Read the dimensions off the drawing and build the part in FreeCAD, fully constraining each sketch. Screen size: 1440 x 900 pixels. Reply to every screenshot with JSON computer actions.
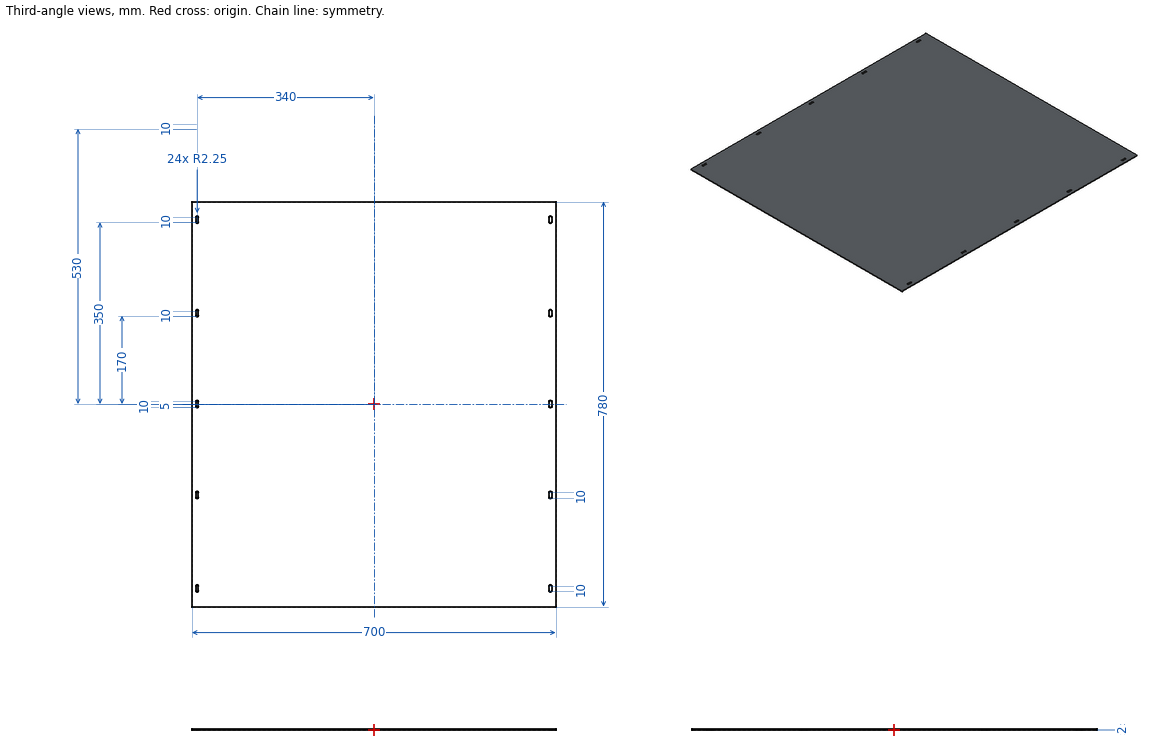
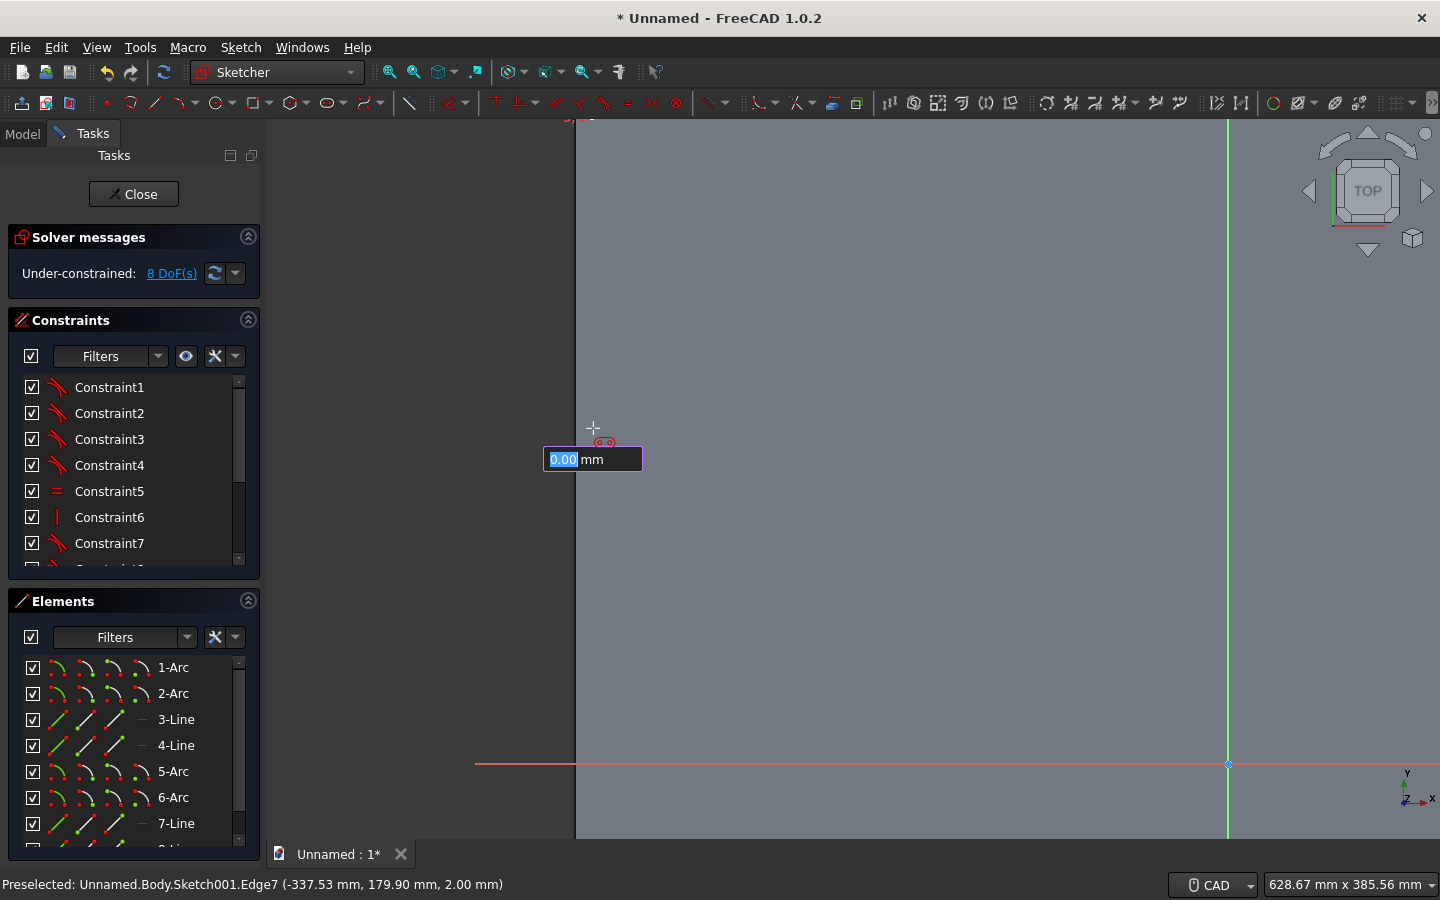
{"action": "scroll", "coordinate": [589, 437], "scroll_direction": "up", "scroll_amount": 7}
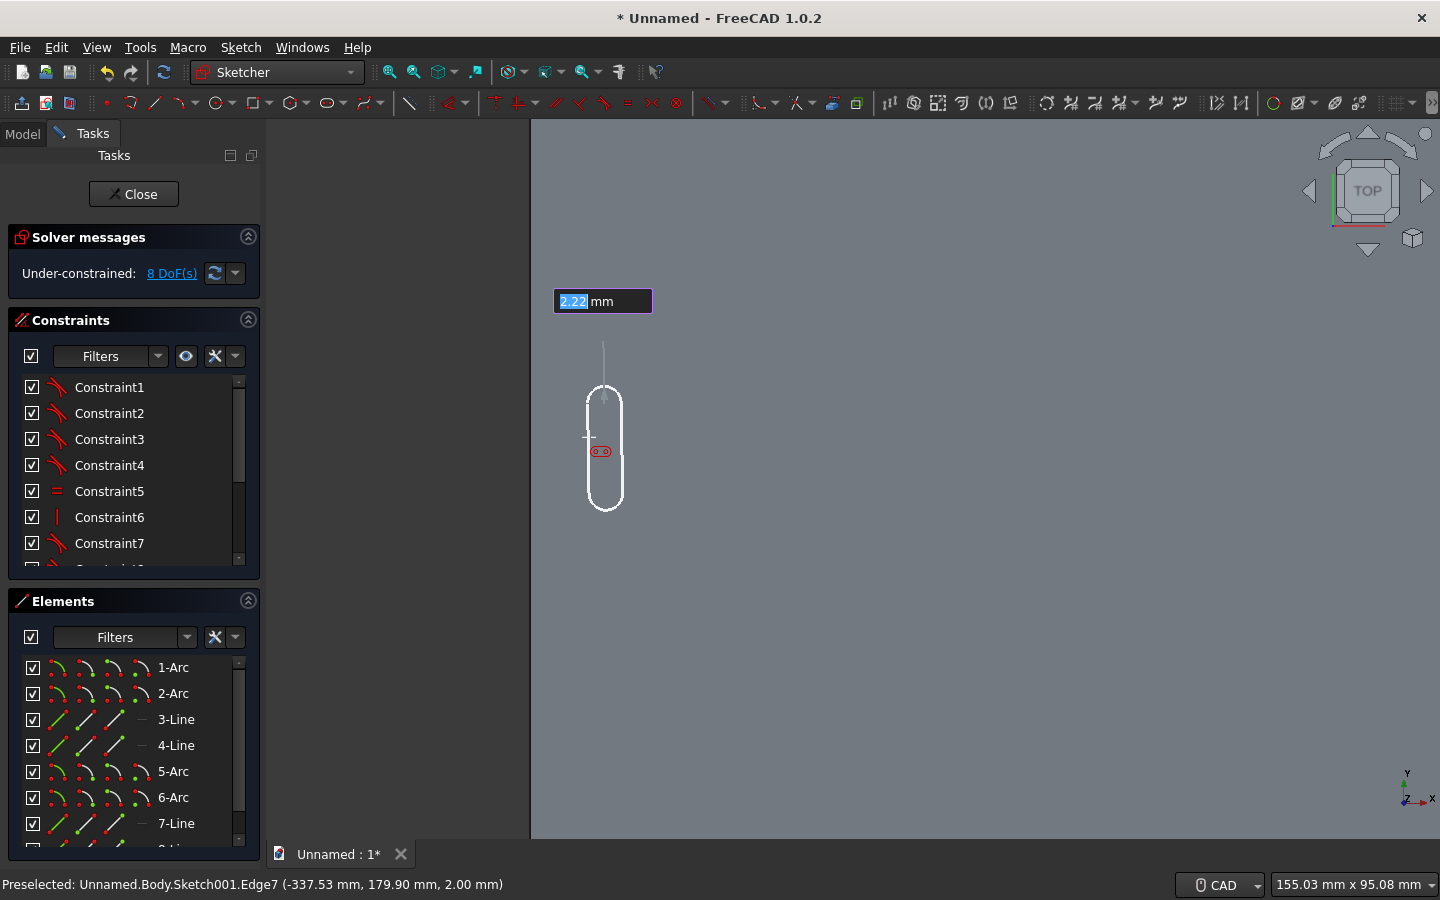
{"action": "left_click", "coordinate": [589, 438]}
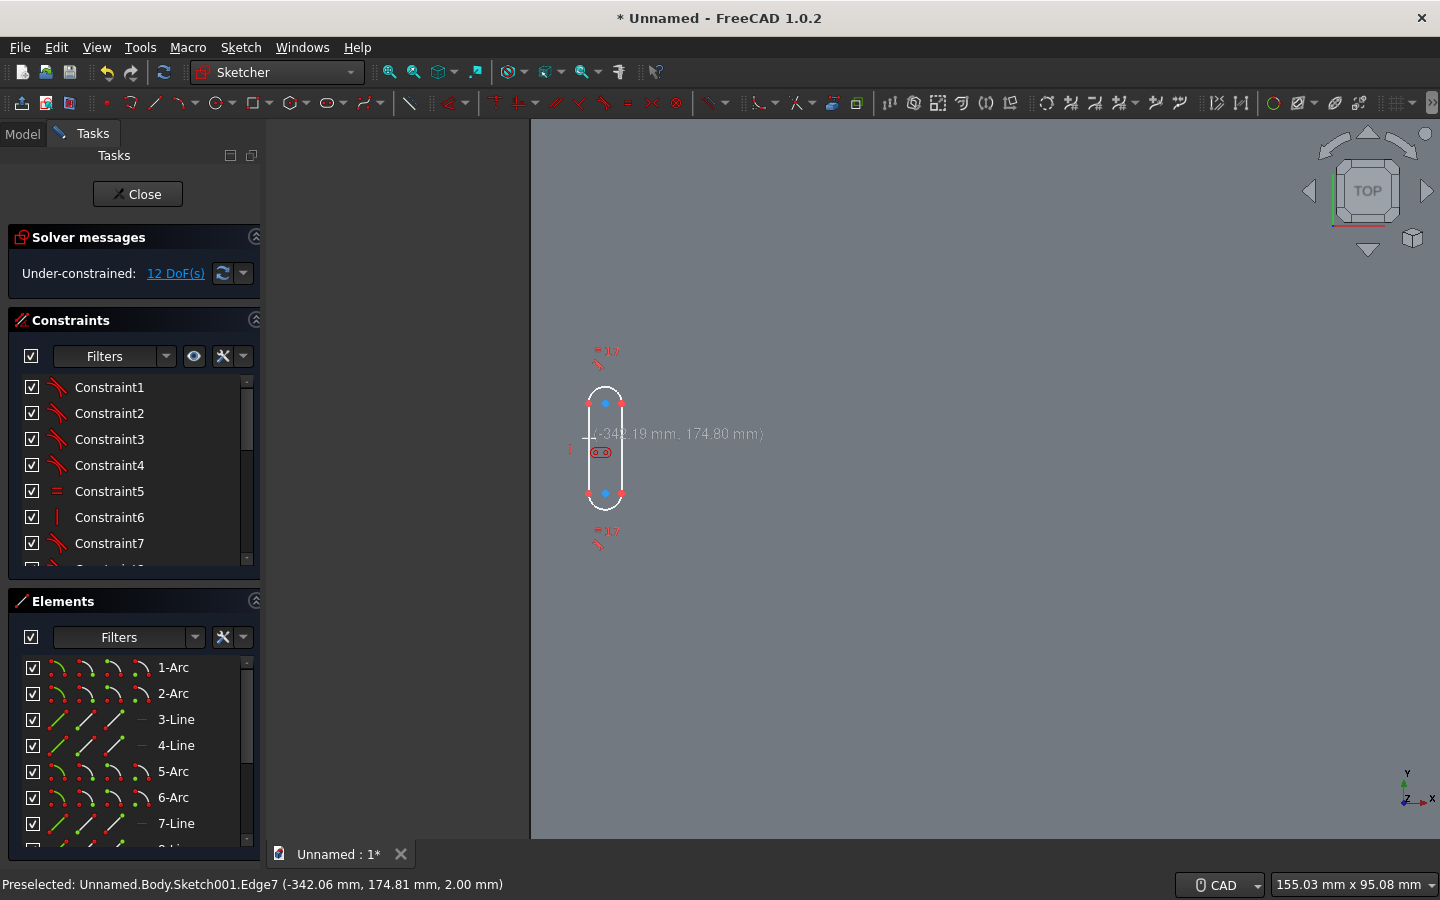
{"action": "scroll", "coordinate": [592, 431], "scroll_direction": "down", "scroll_amount": 13}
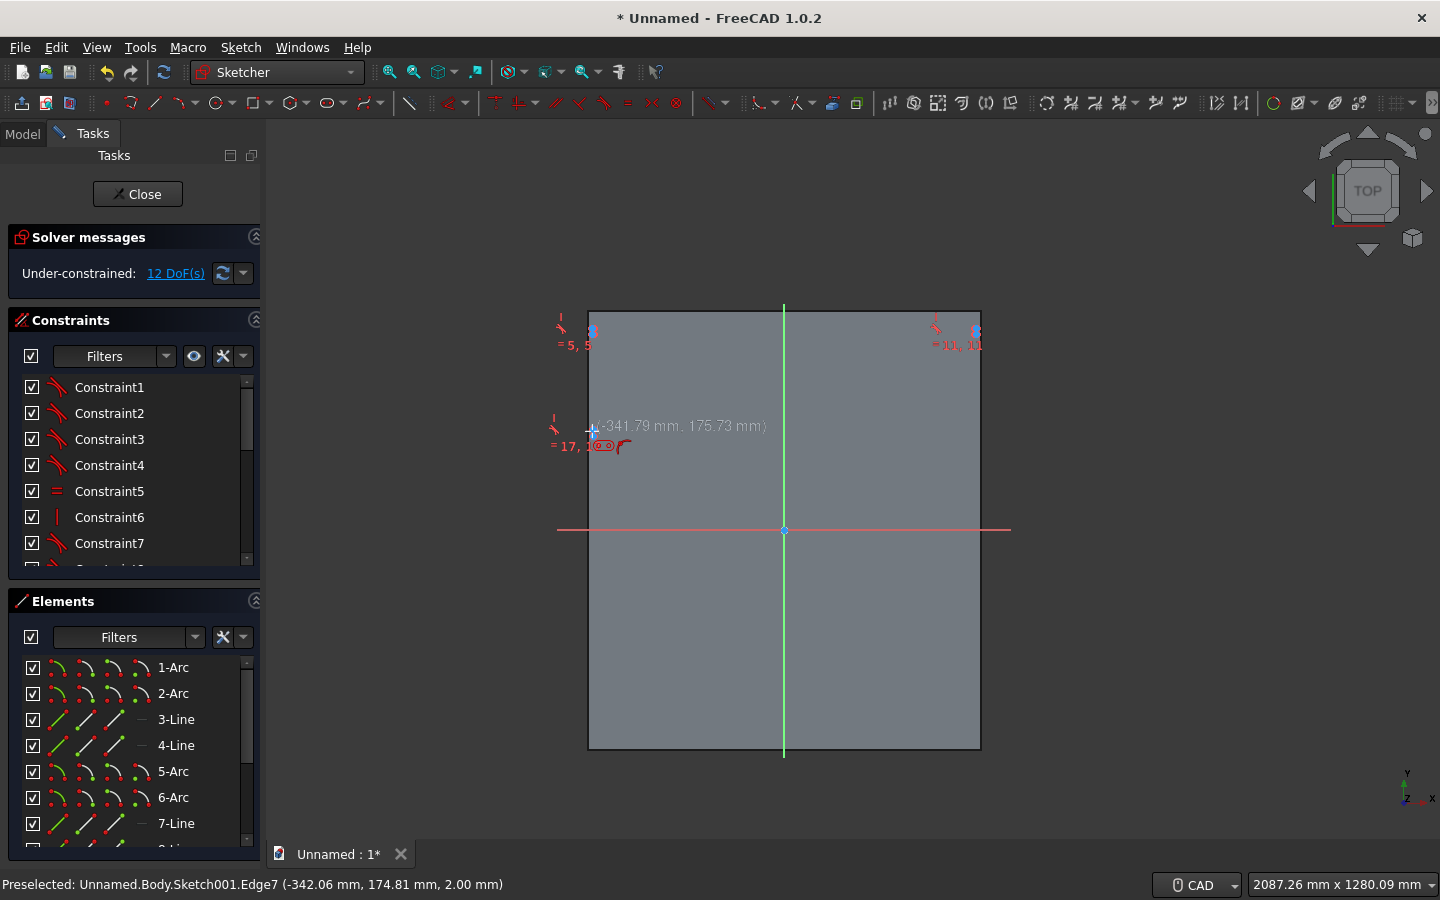
{"action": "scroll", "coordinate": [593, 533], "scroll_direction": "up", "scroll_amount": 15}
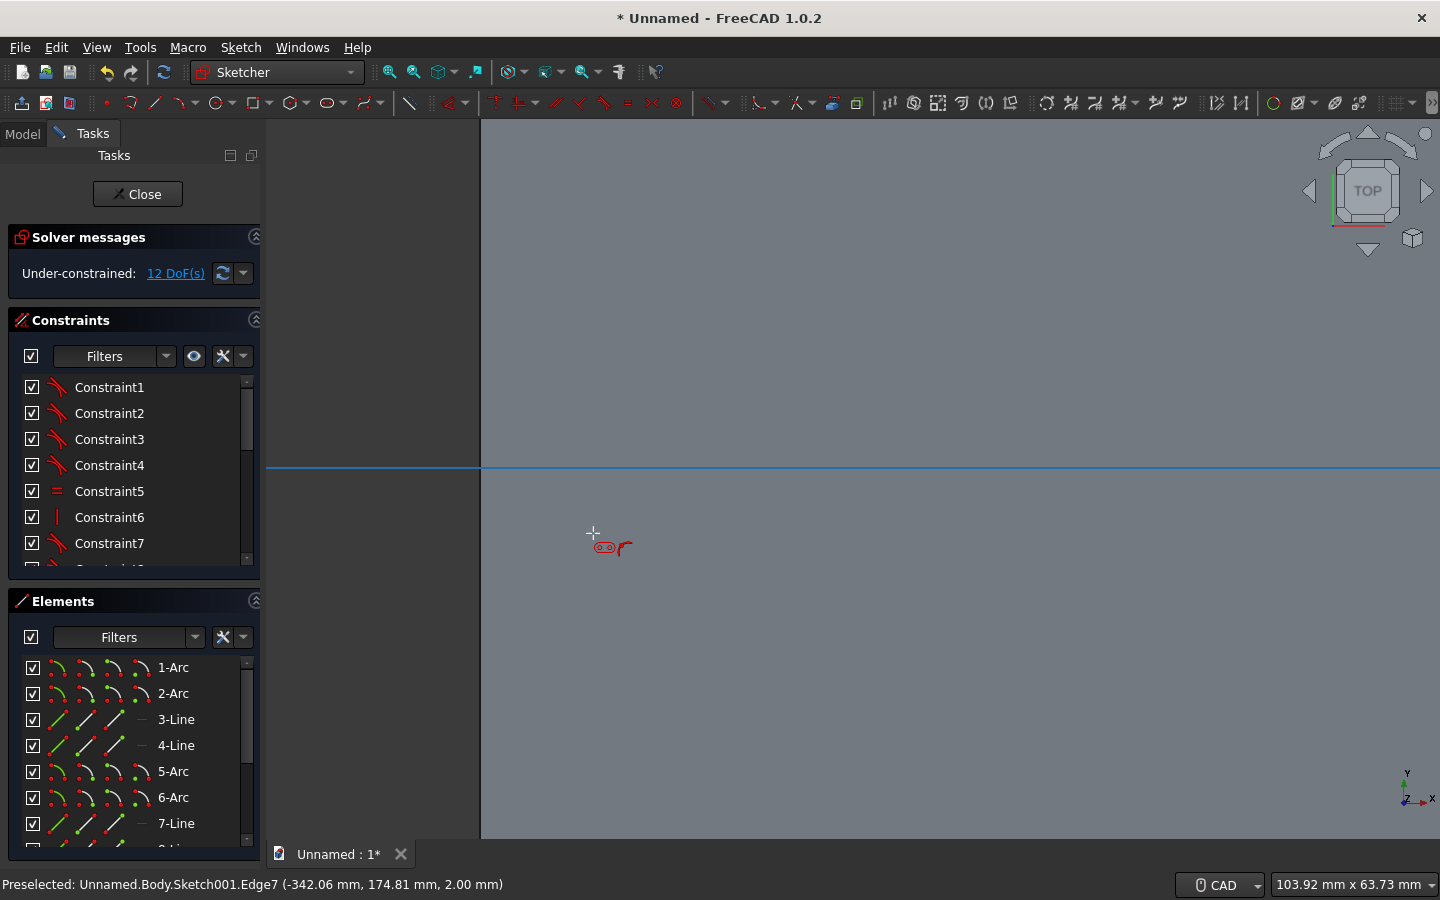
{"action": "scroll", "coordinate": [593, 533], "scroll_direction": "down", "scroll_amount": 15}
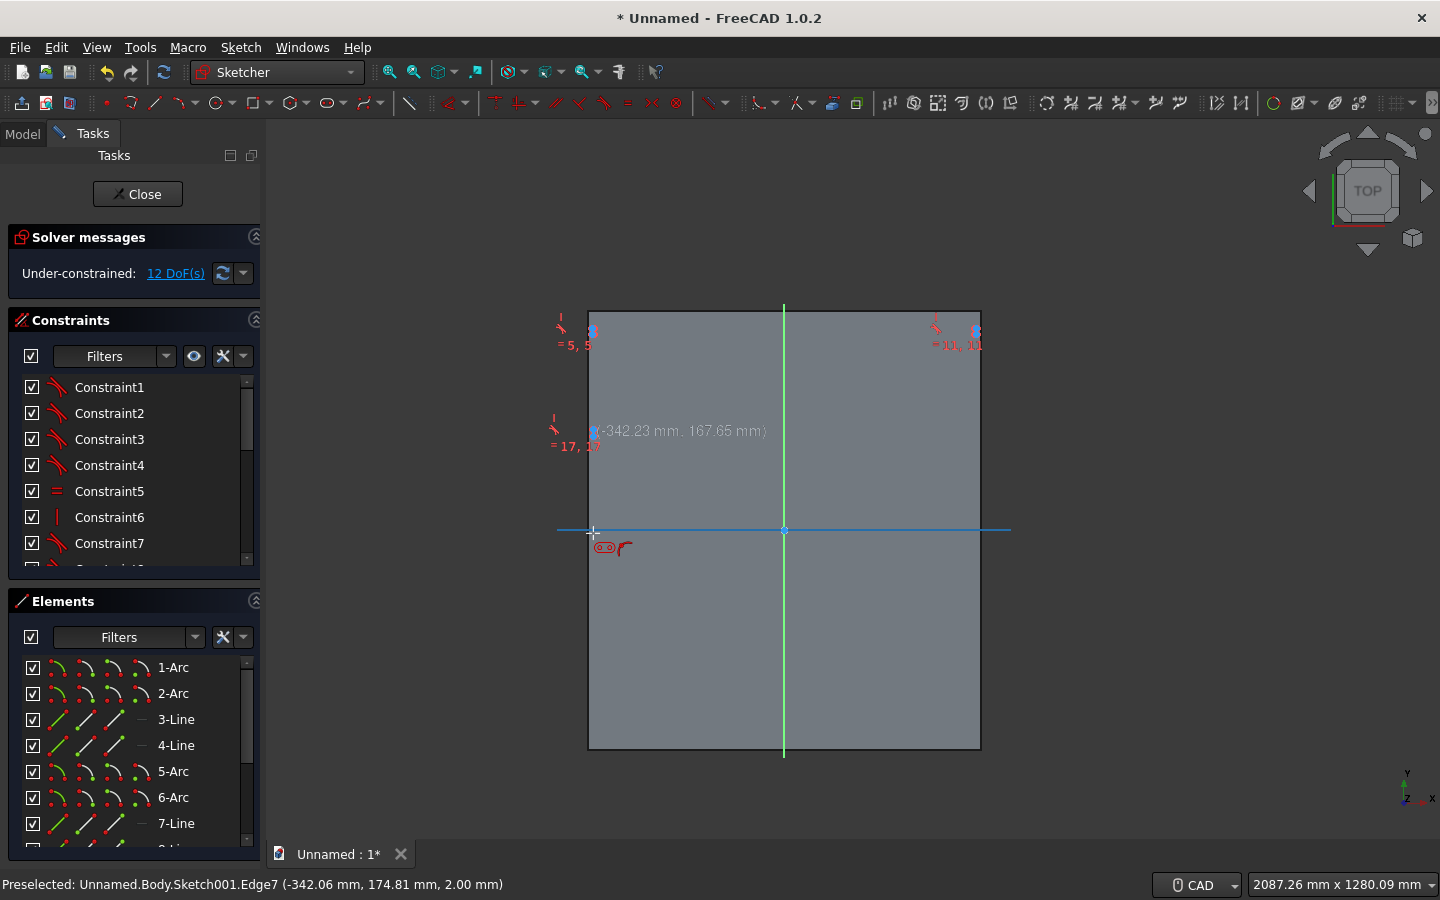
{"action": "scroll", "coordinate": [593, 533], "scroll_direction": "up", "scroll_amount": 9}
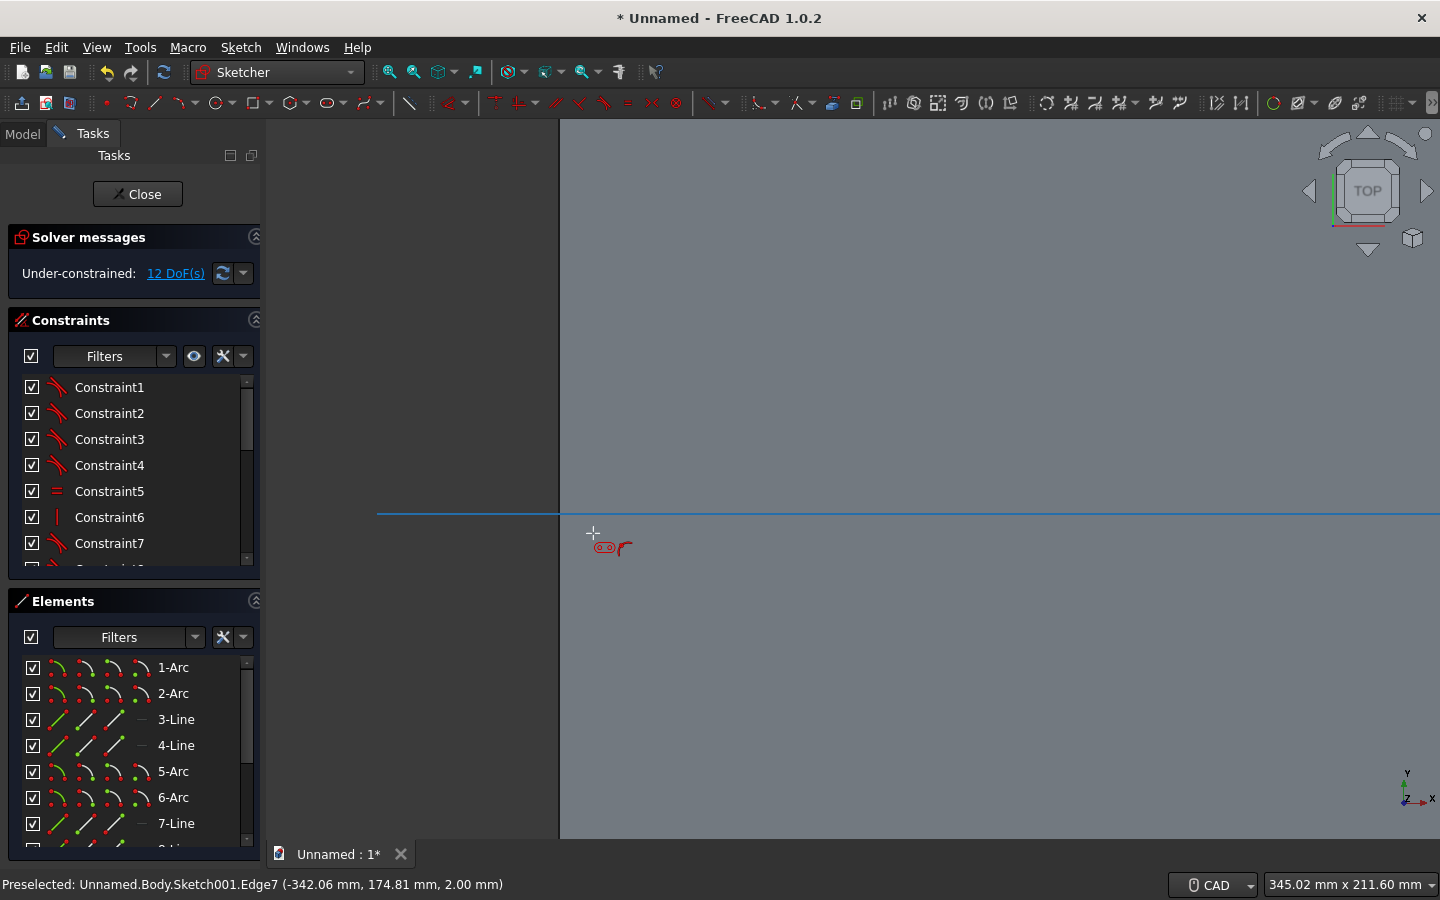
{"action": "left_click", "coordinate": [593, 531]}